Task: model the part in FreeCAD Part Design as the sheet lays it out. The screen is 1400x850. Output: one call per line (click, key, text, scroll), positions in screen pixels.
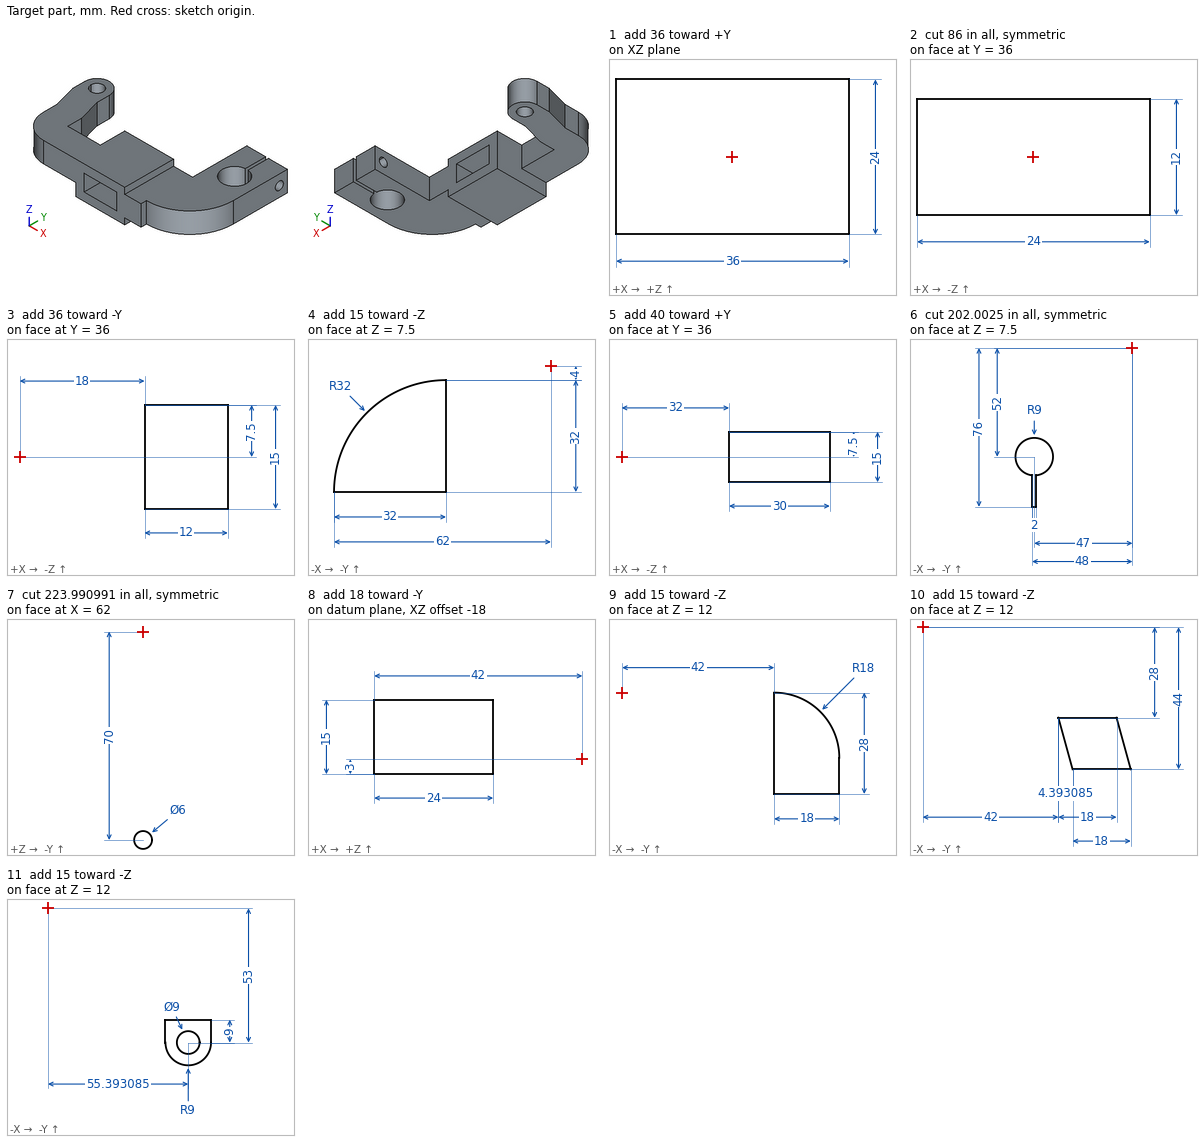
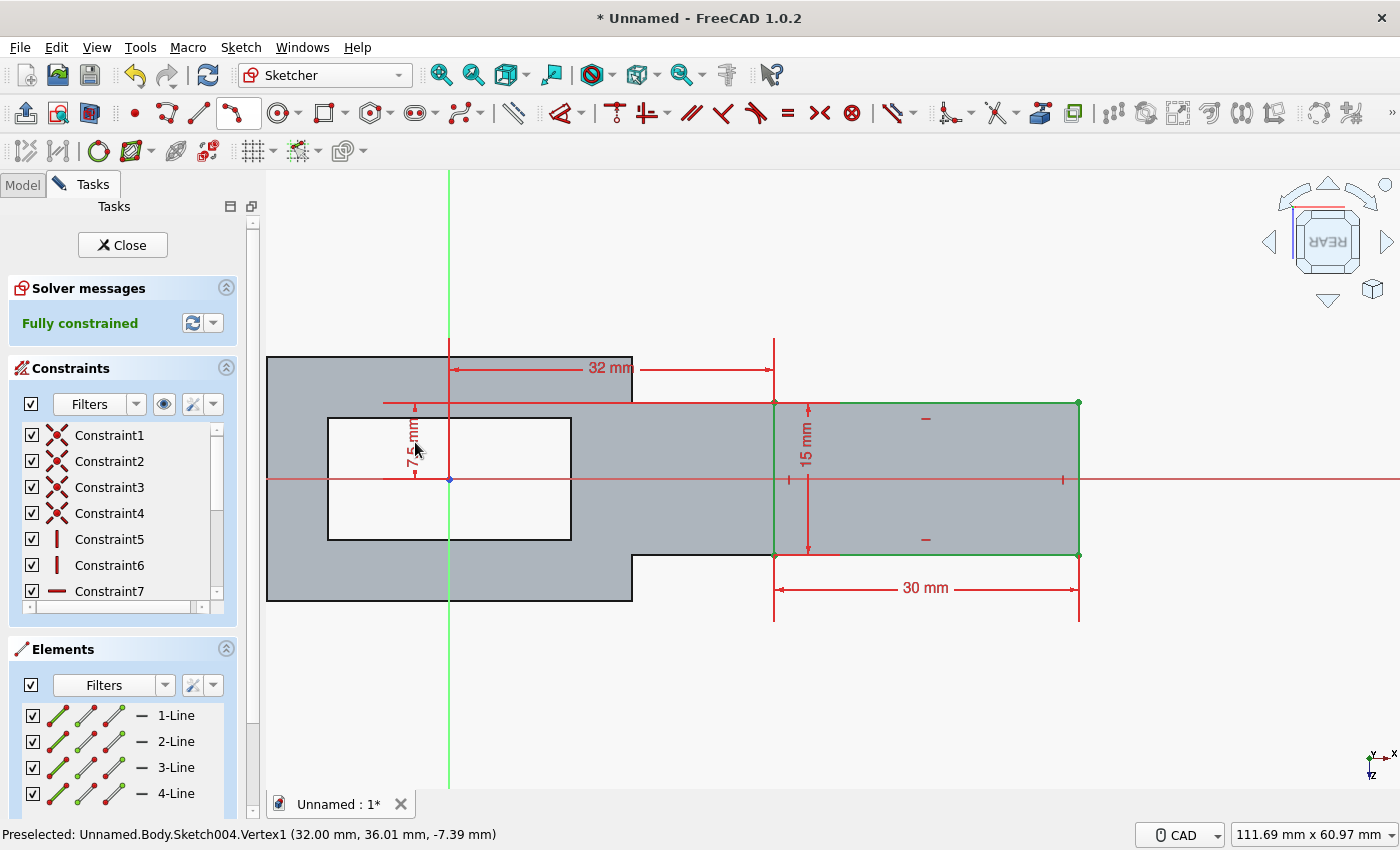
click(123, 245)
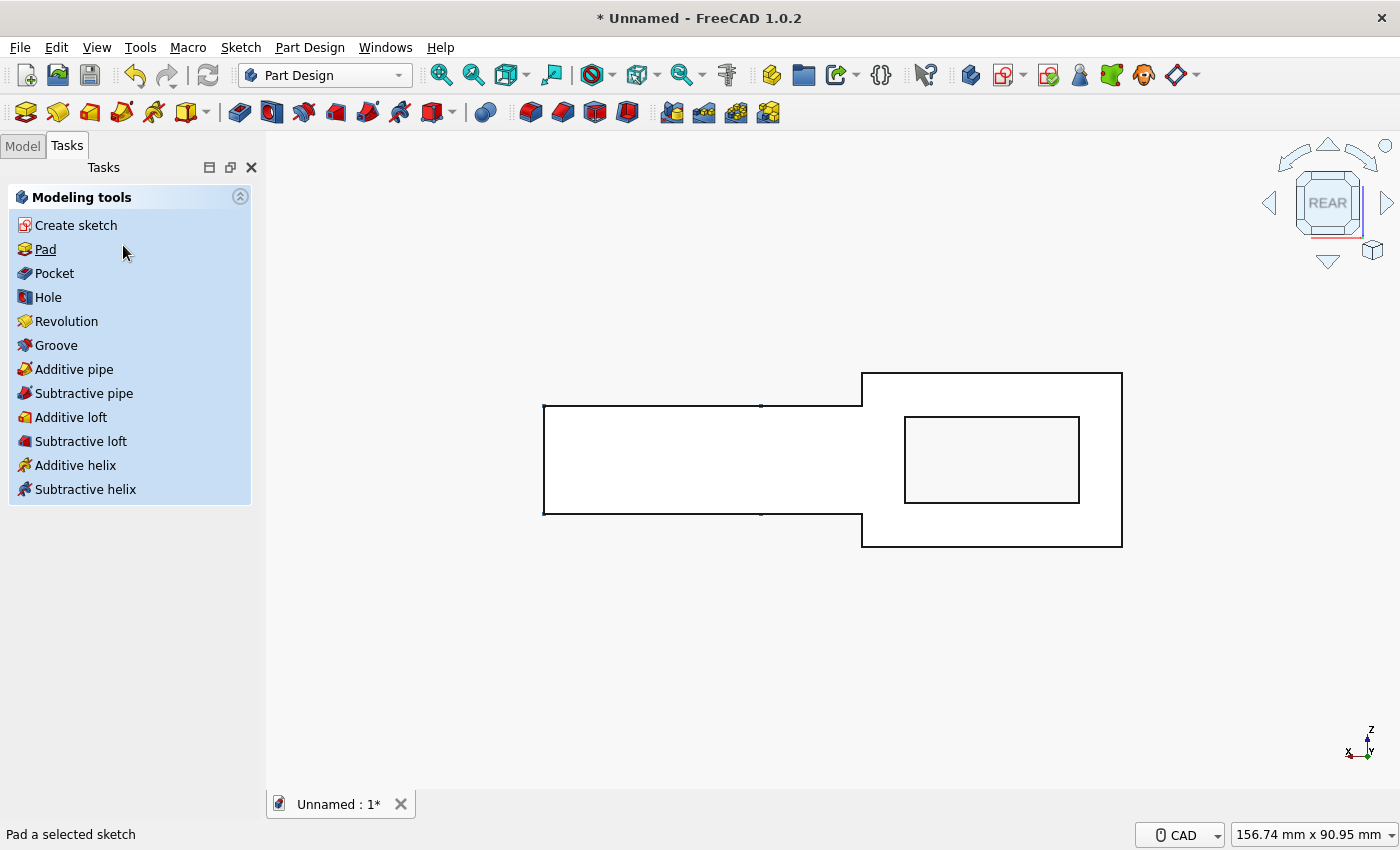
click(26, 112)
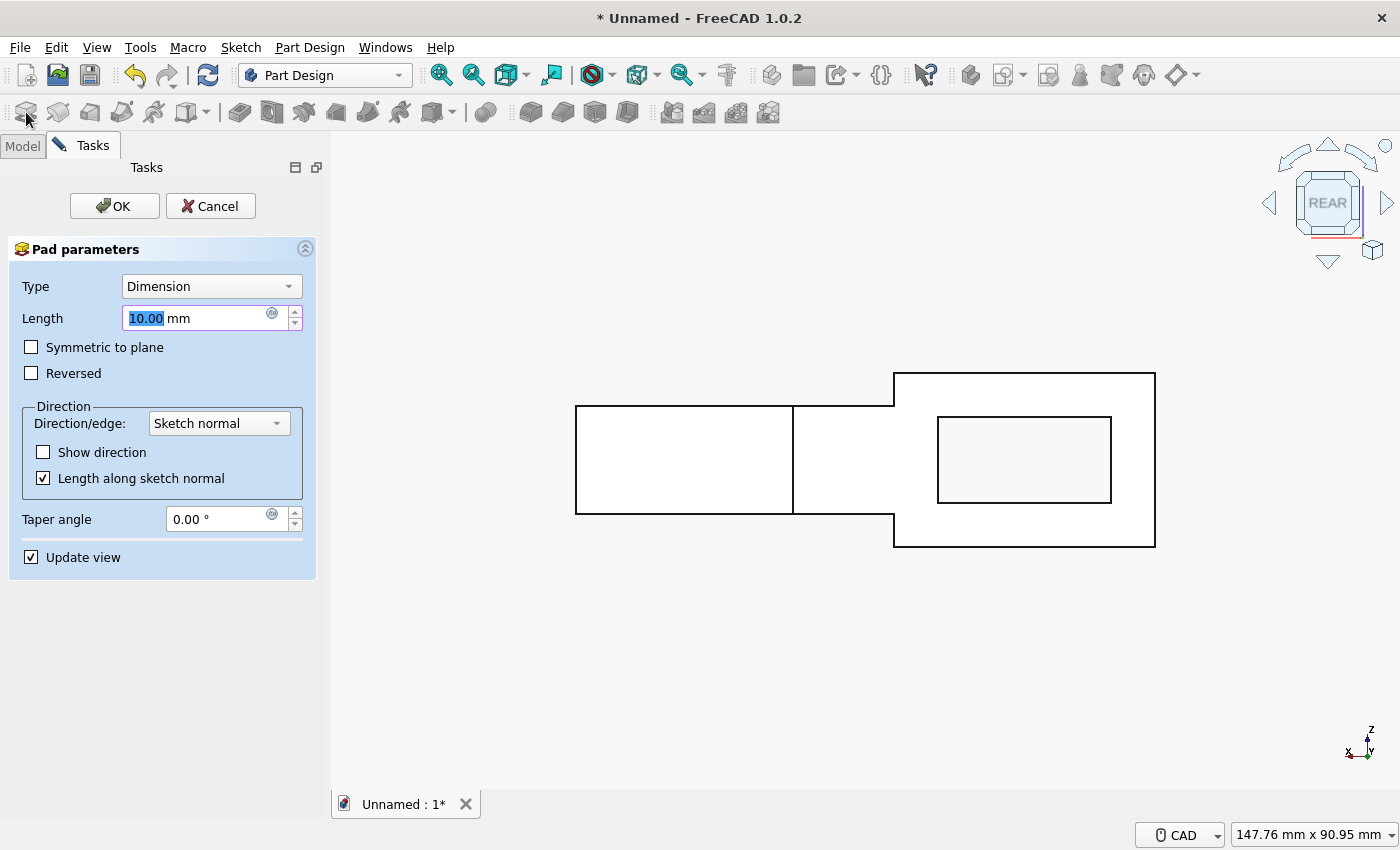
text(40)
key(Tab)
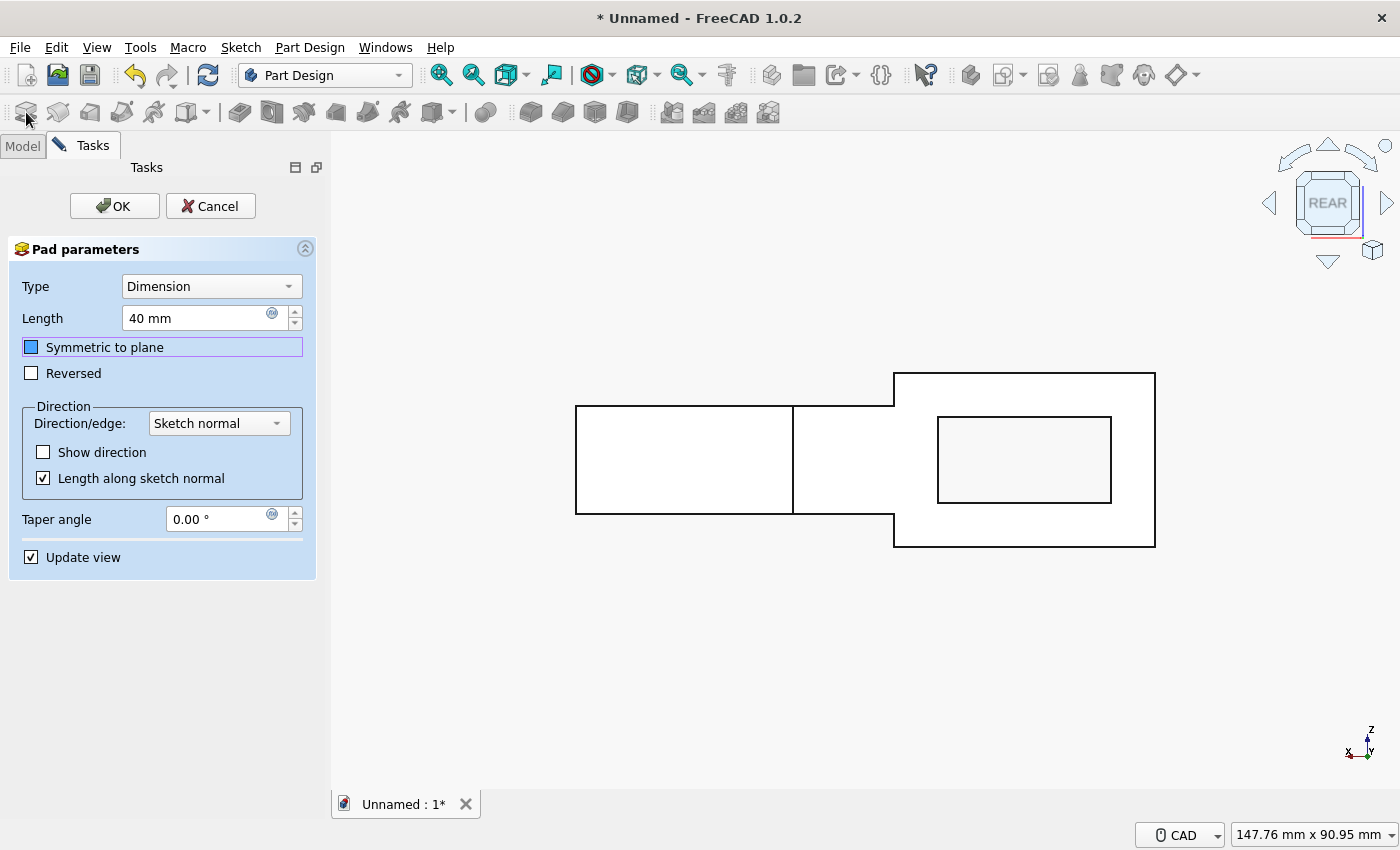
click(115, 206)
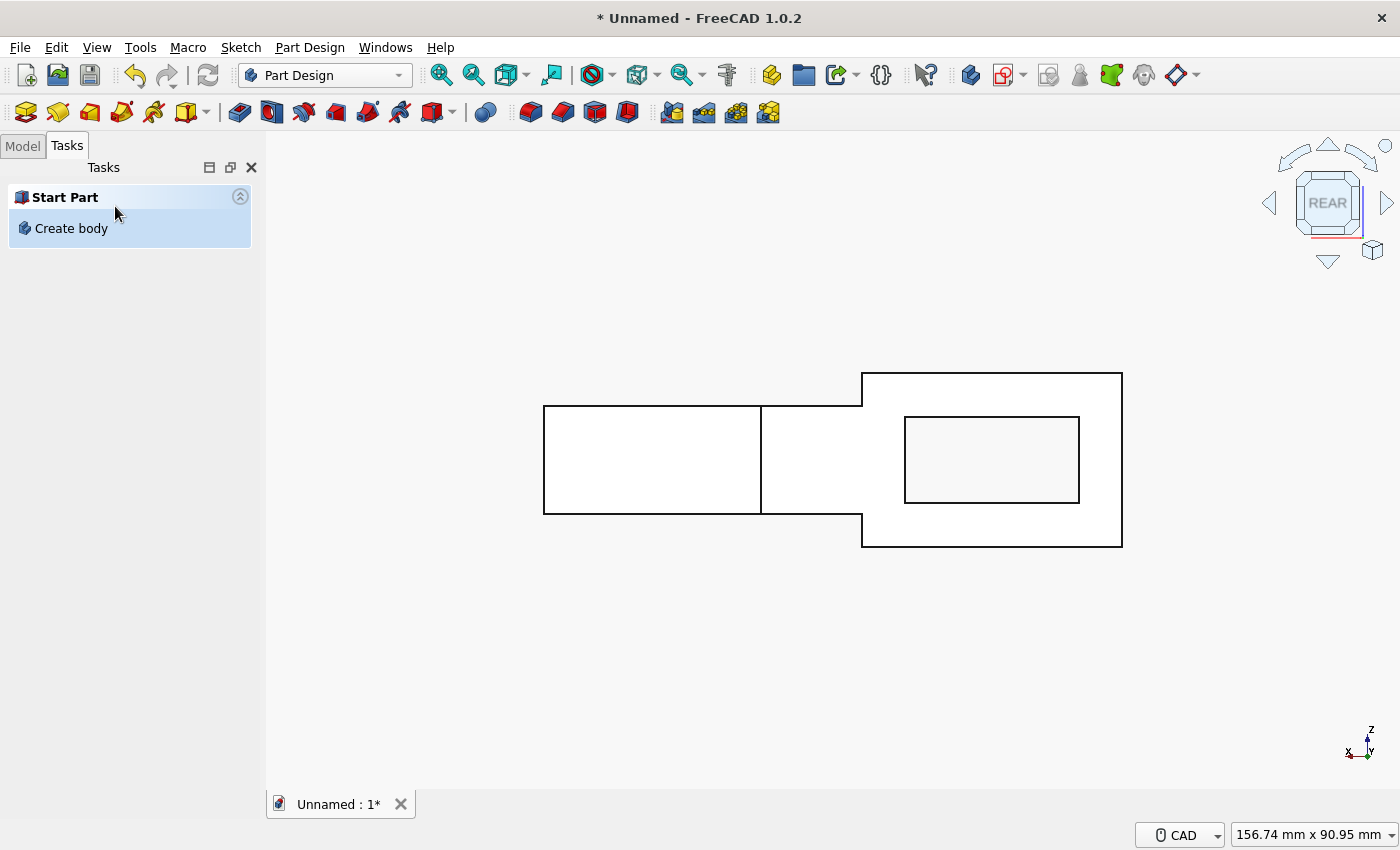
key(0)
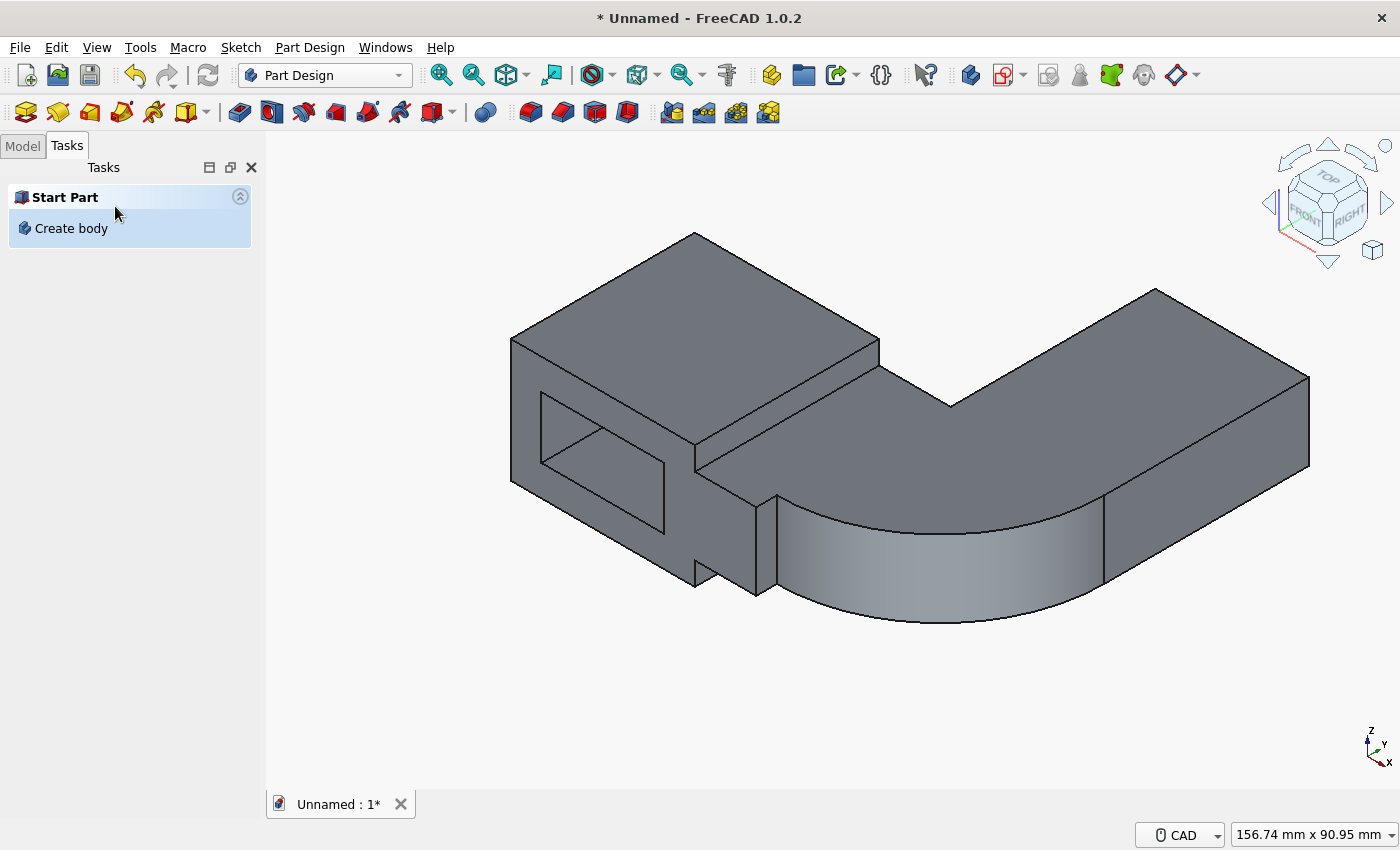
key(v)
key(f)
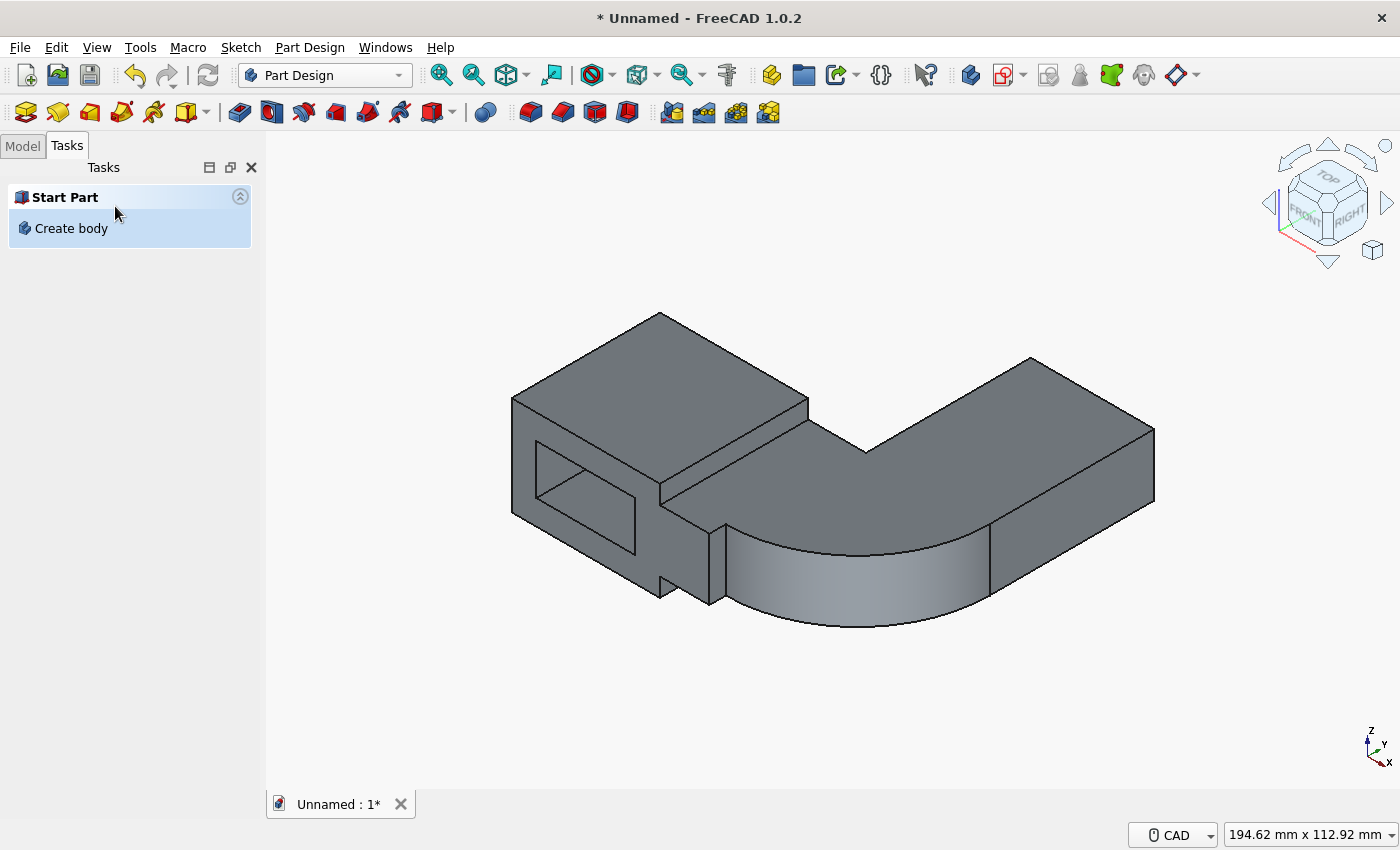
click(1023, 429)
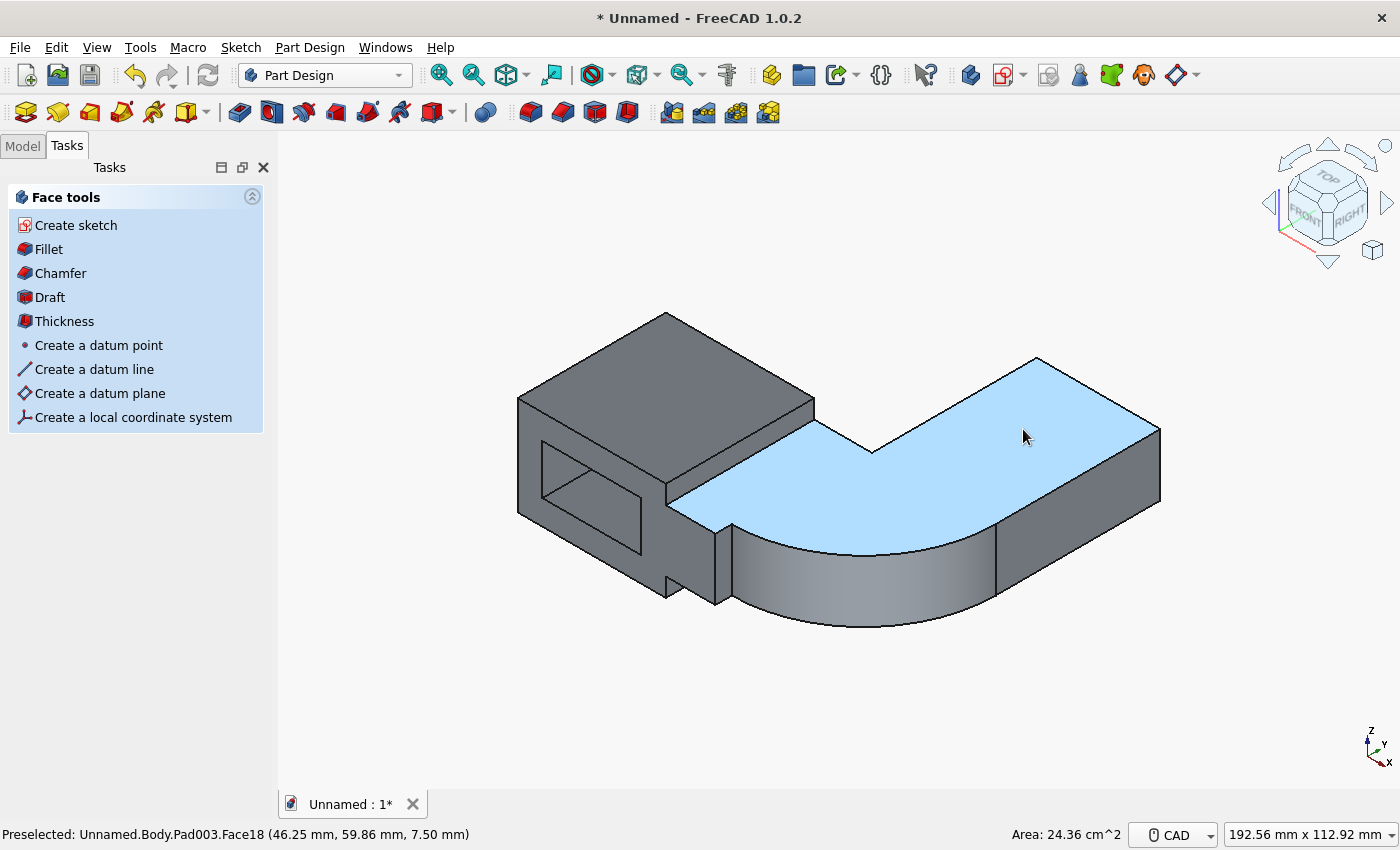
click(1004, 76)